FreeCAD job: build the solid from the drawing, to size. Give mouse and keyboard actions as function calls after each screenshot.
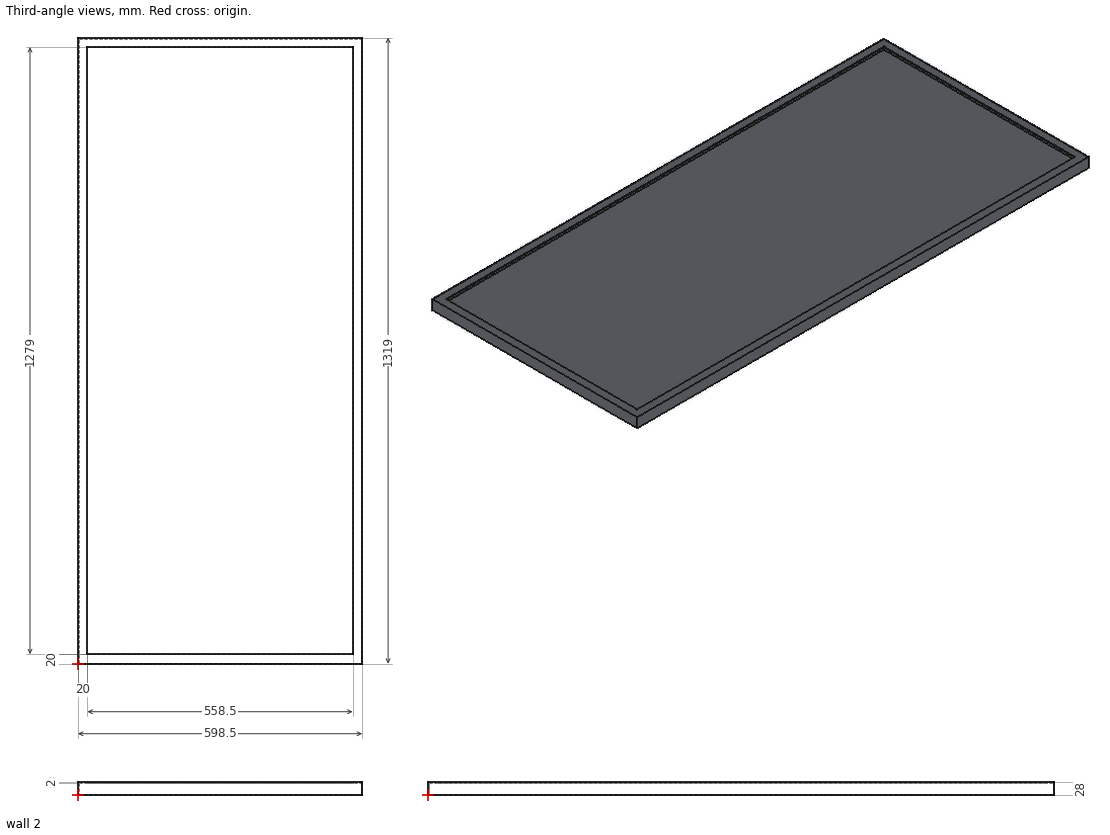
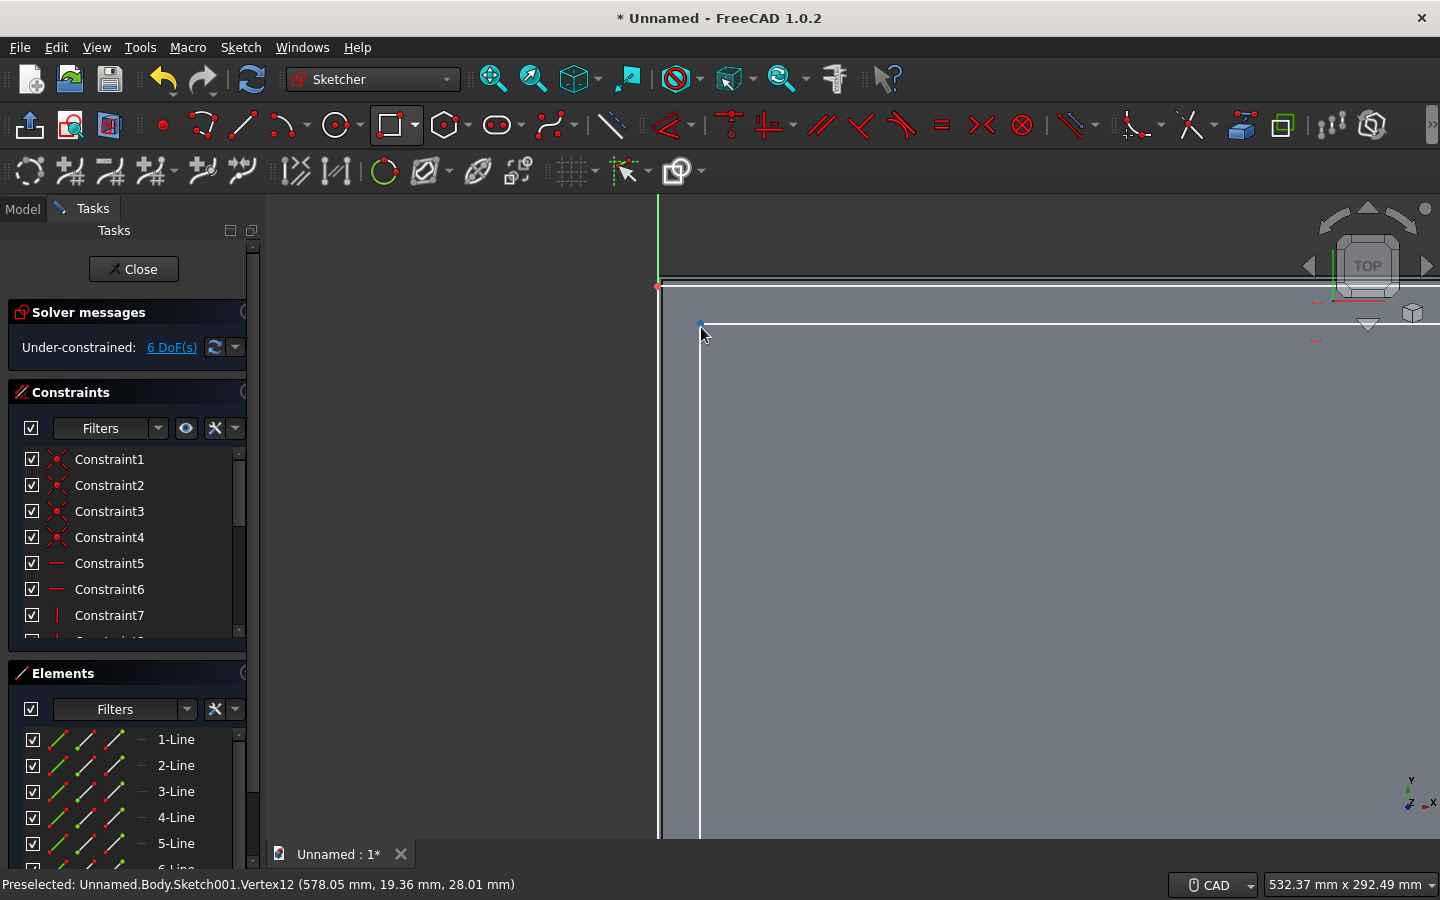
click(700, 324)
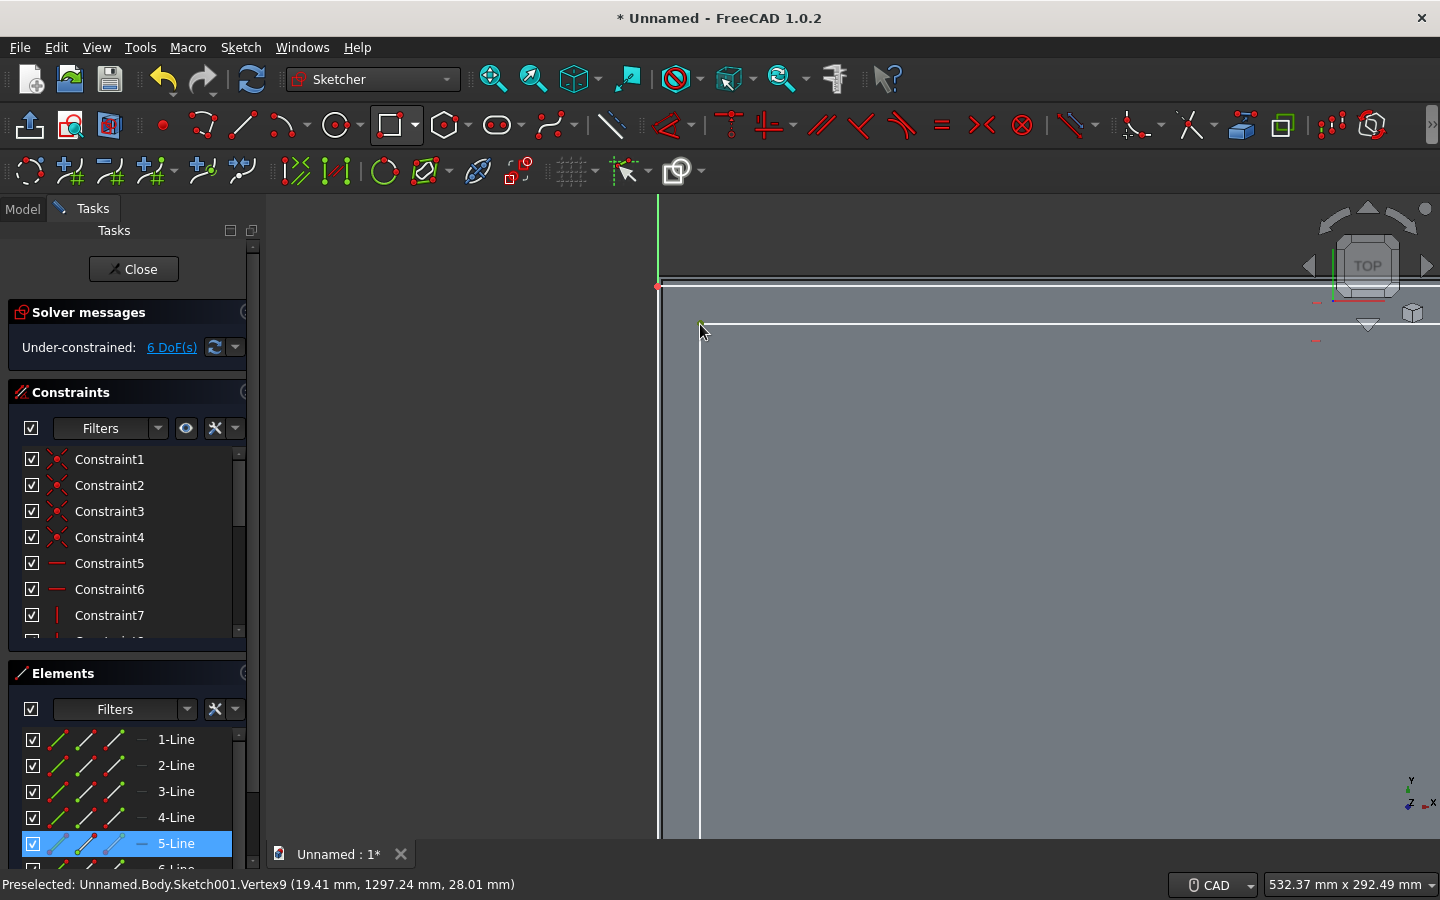
key(l)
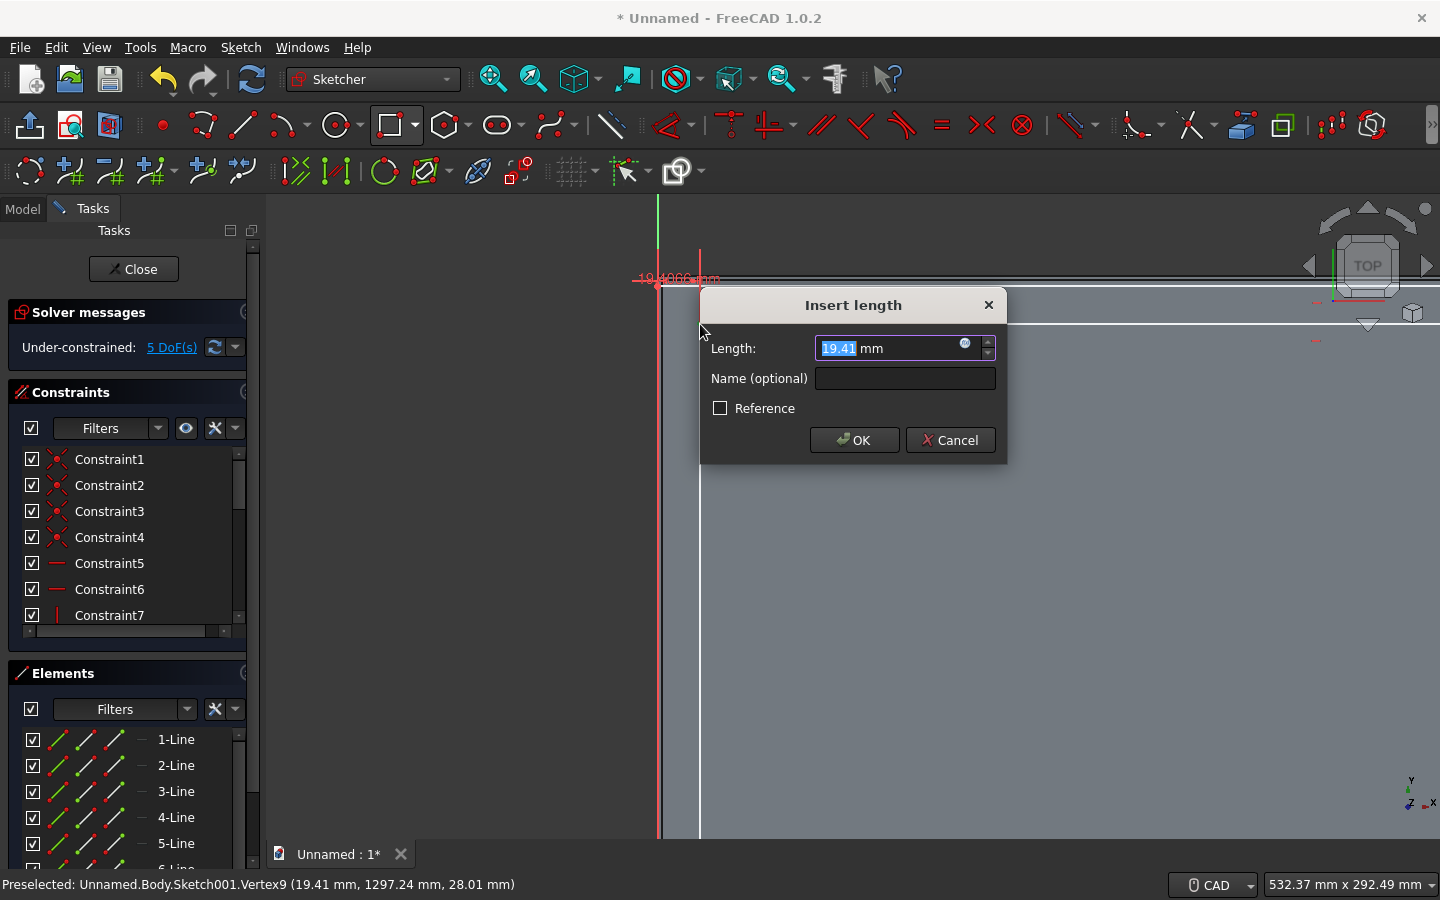
text(20)
key(Return)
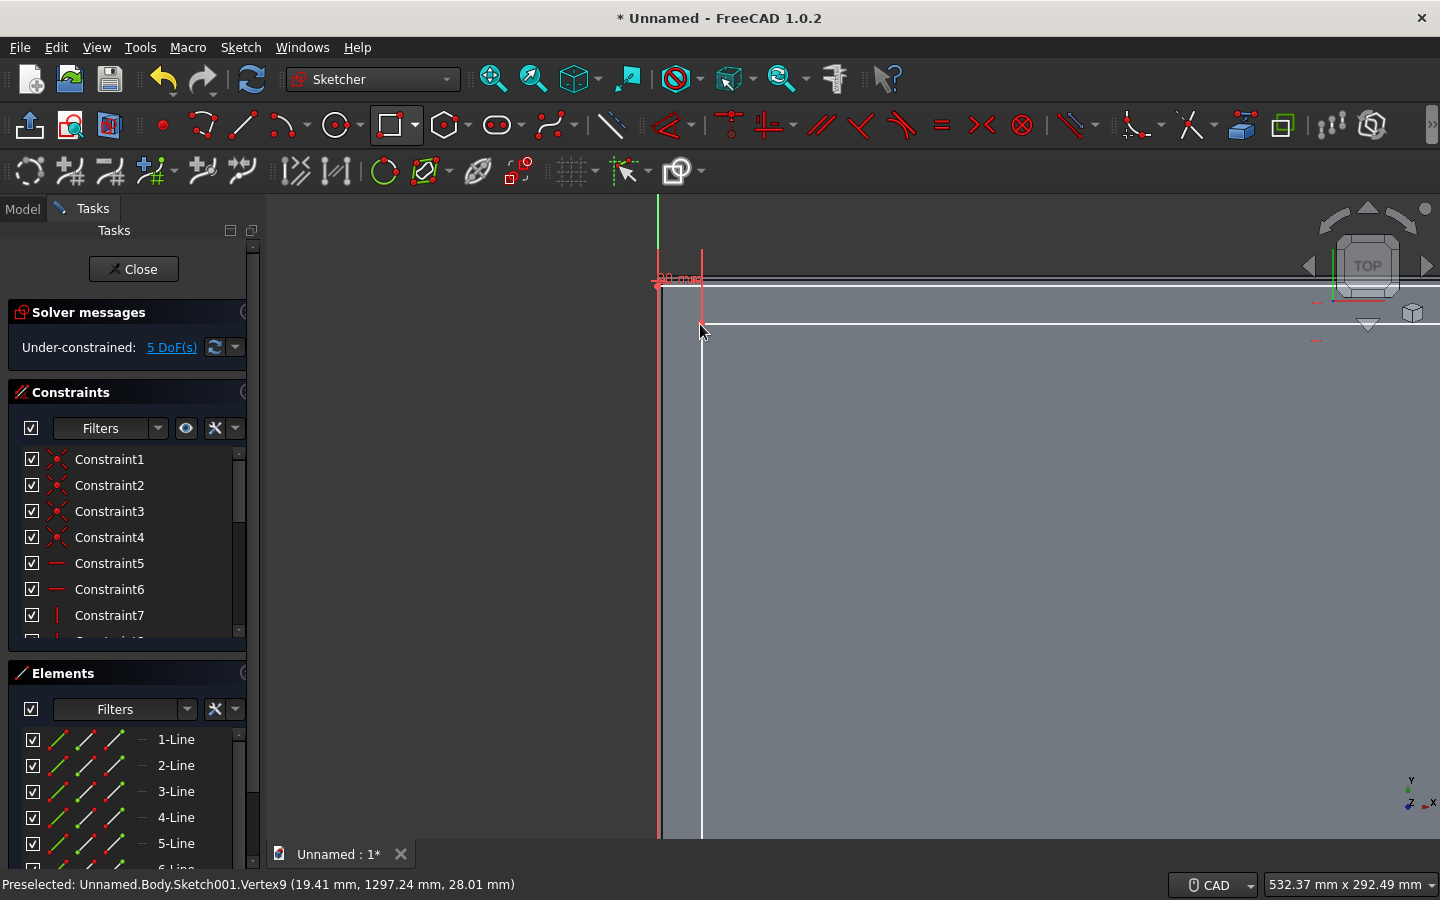
scroll(701, 327, down, 10)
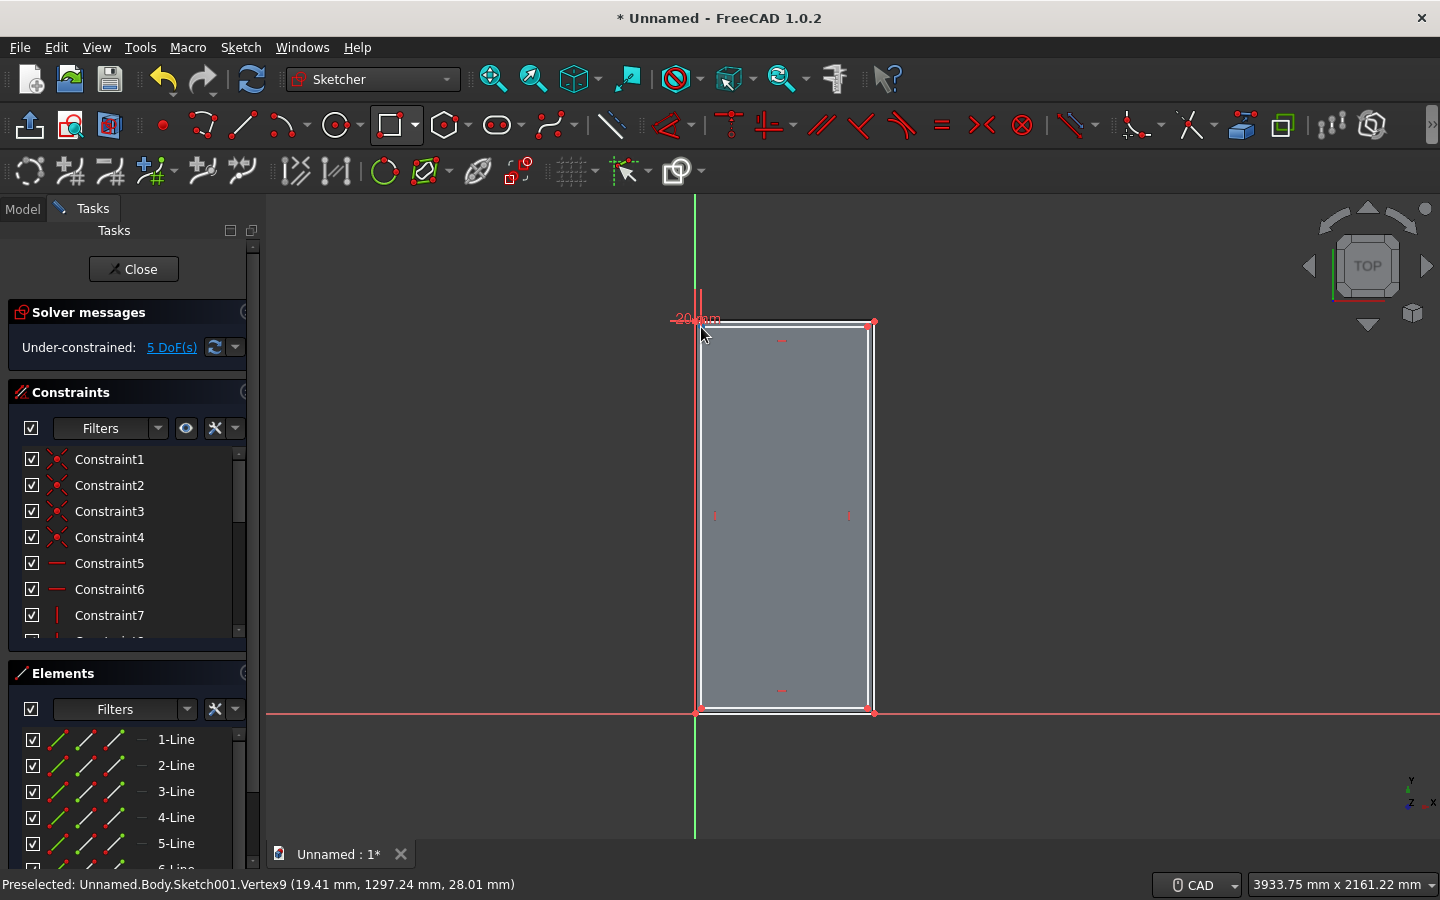
scroll(701, 708, up, 10)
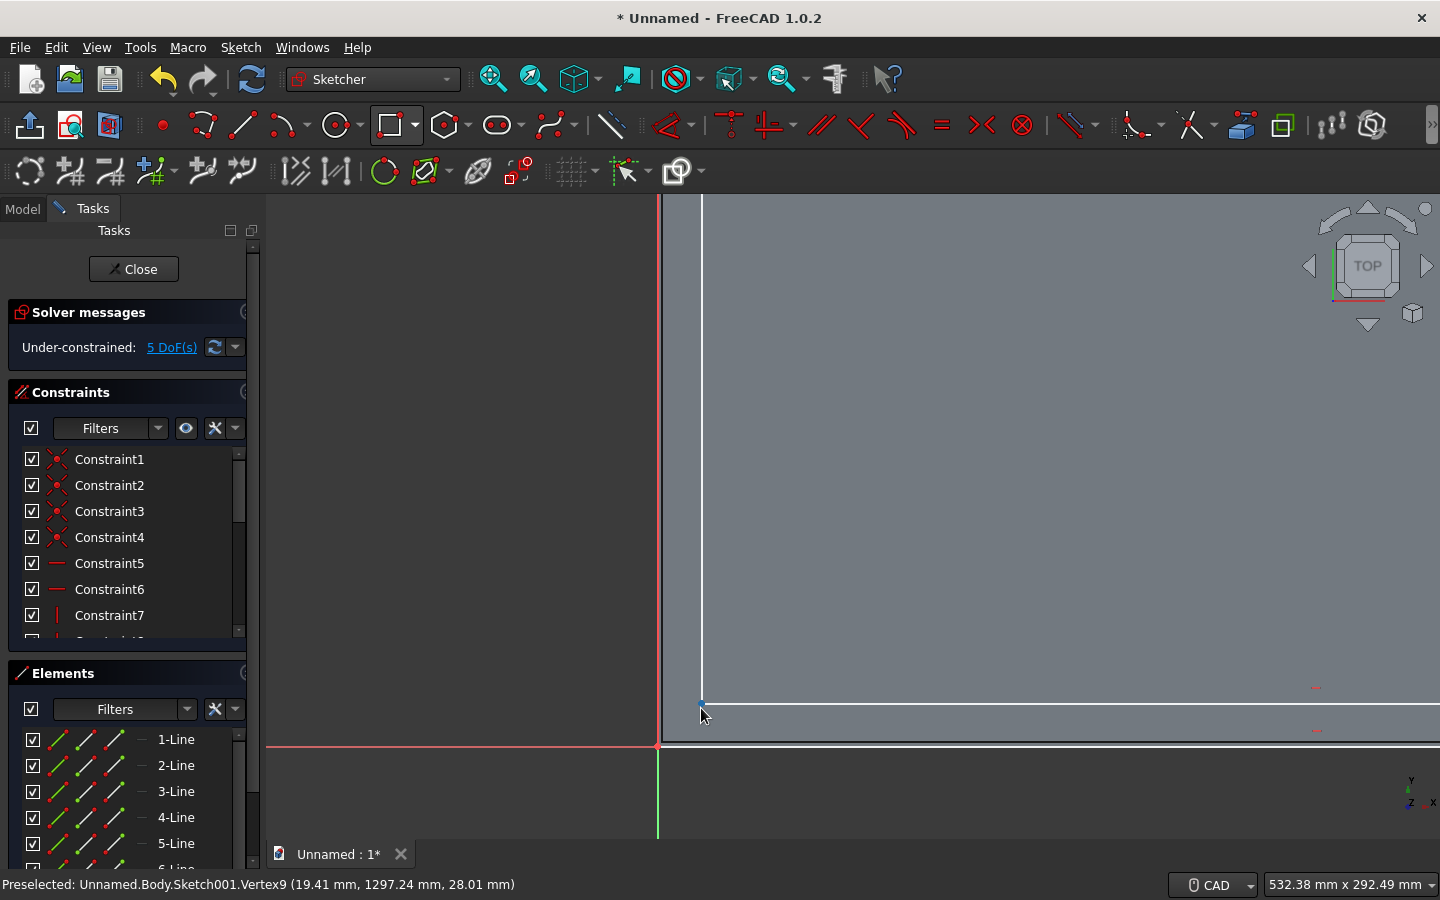
click(702, 704)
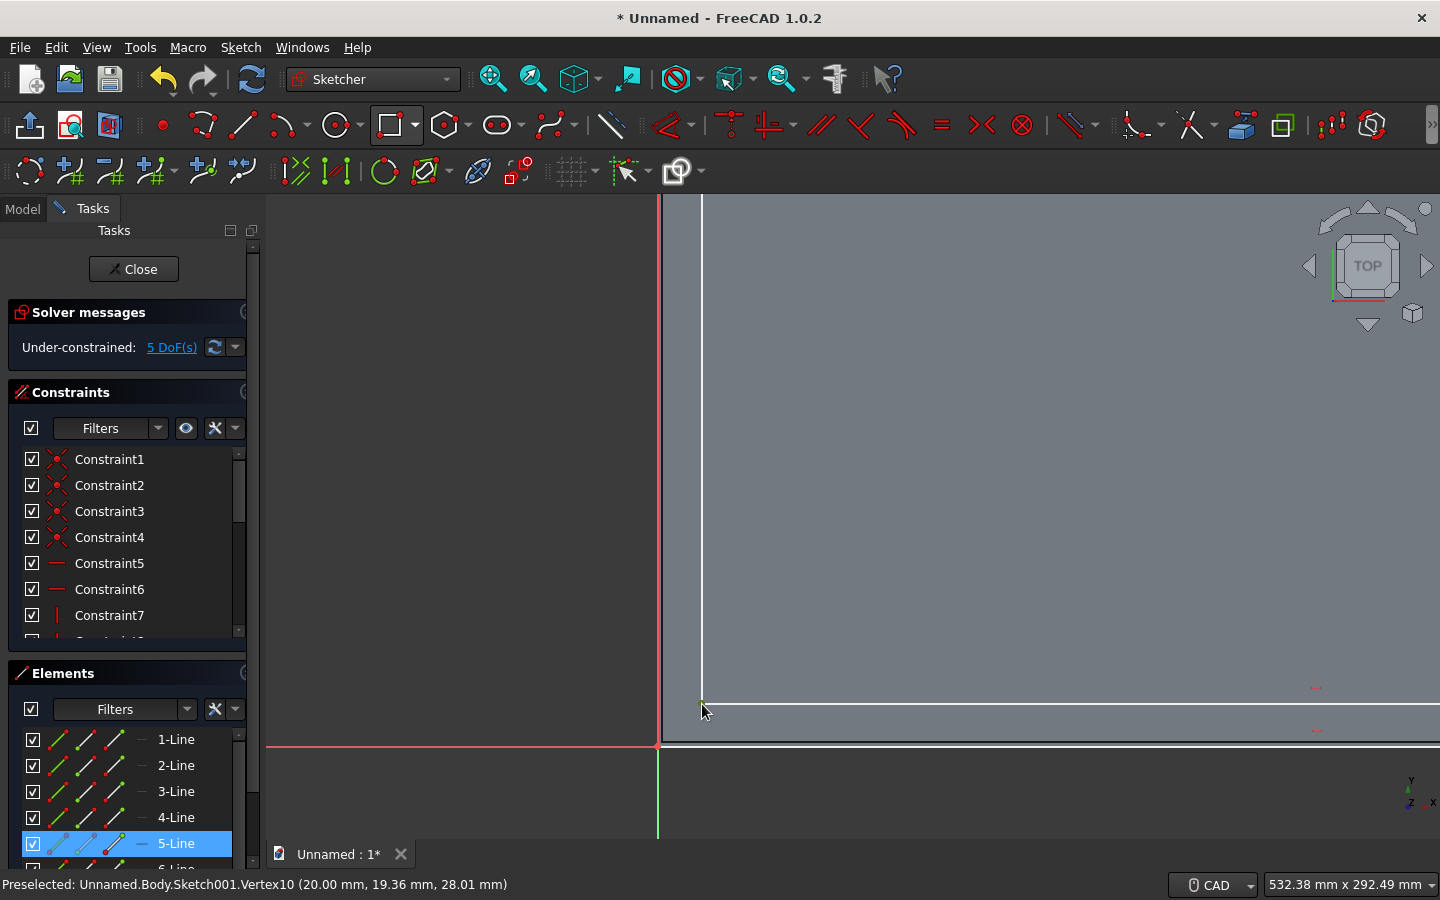
key(i)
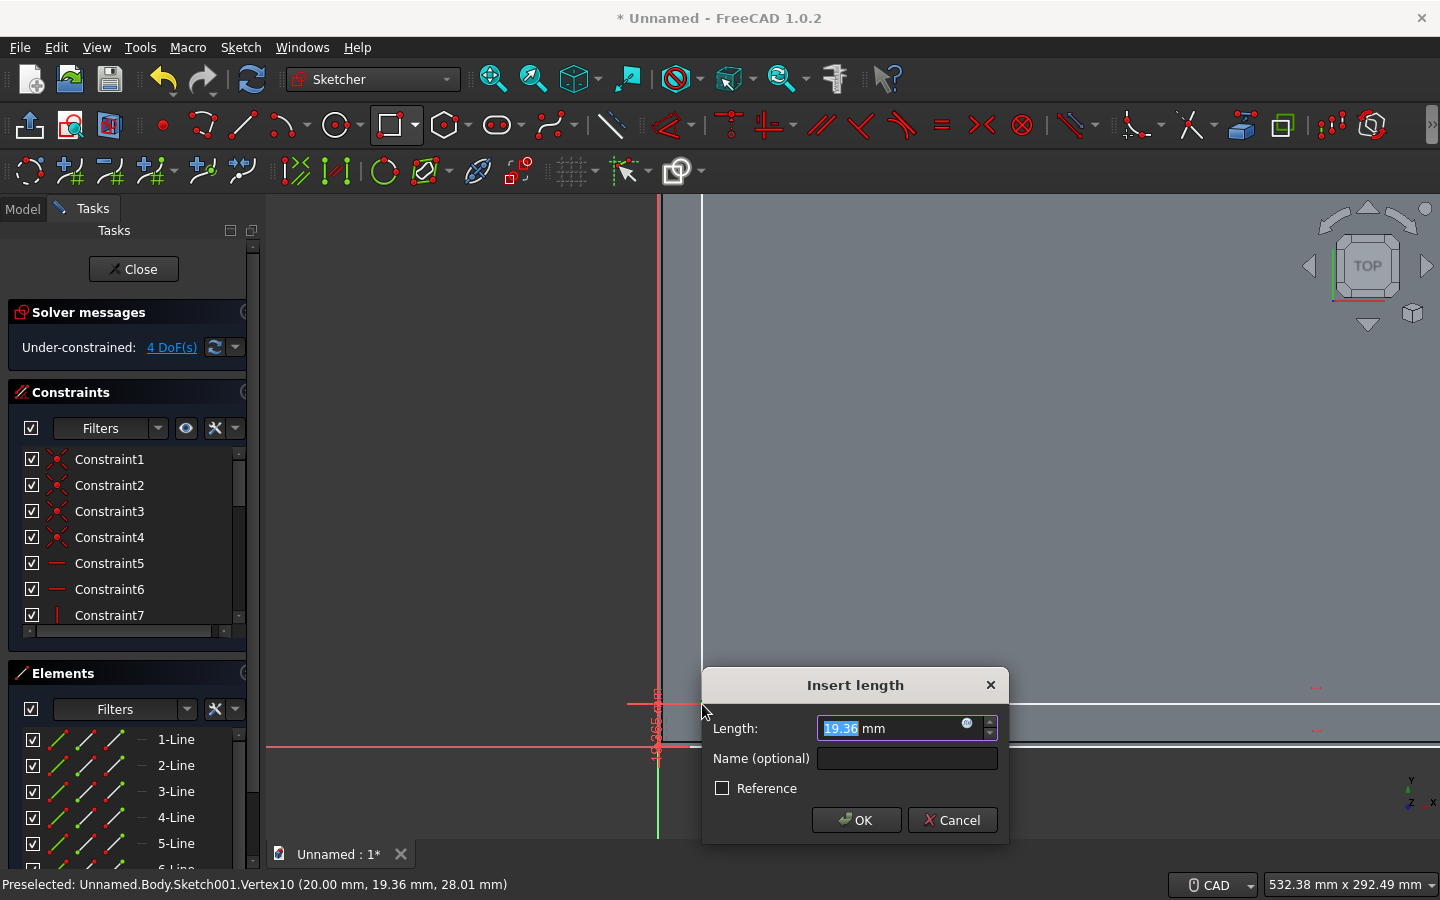
text(20)
key(Return)